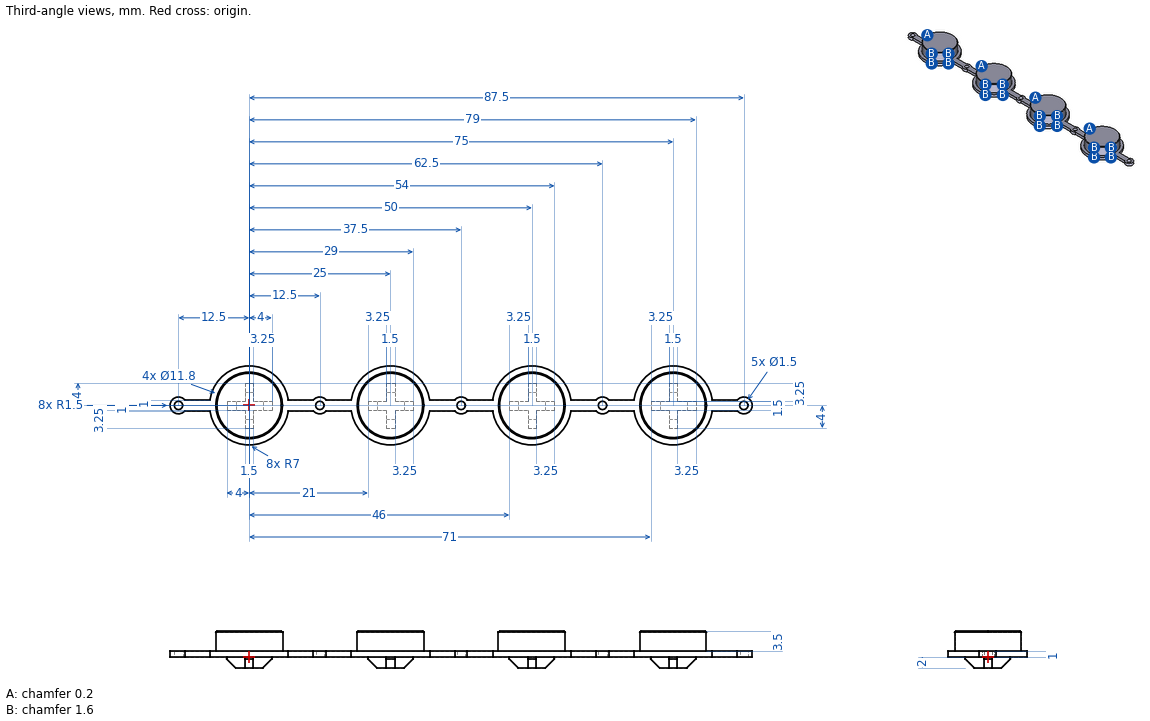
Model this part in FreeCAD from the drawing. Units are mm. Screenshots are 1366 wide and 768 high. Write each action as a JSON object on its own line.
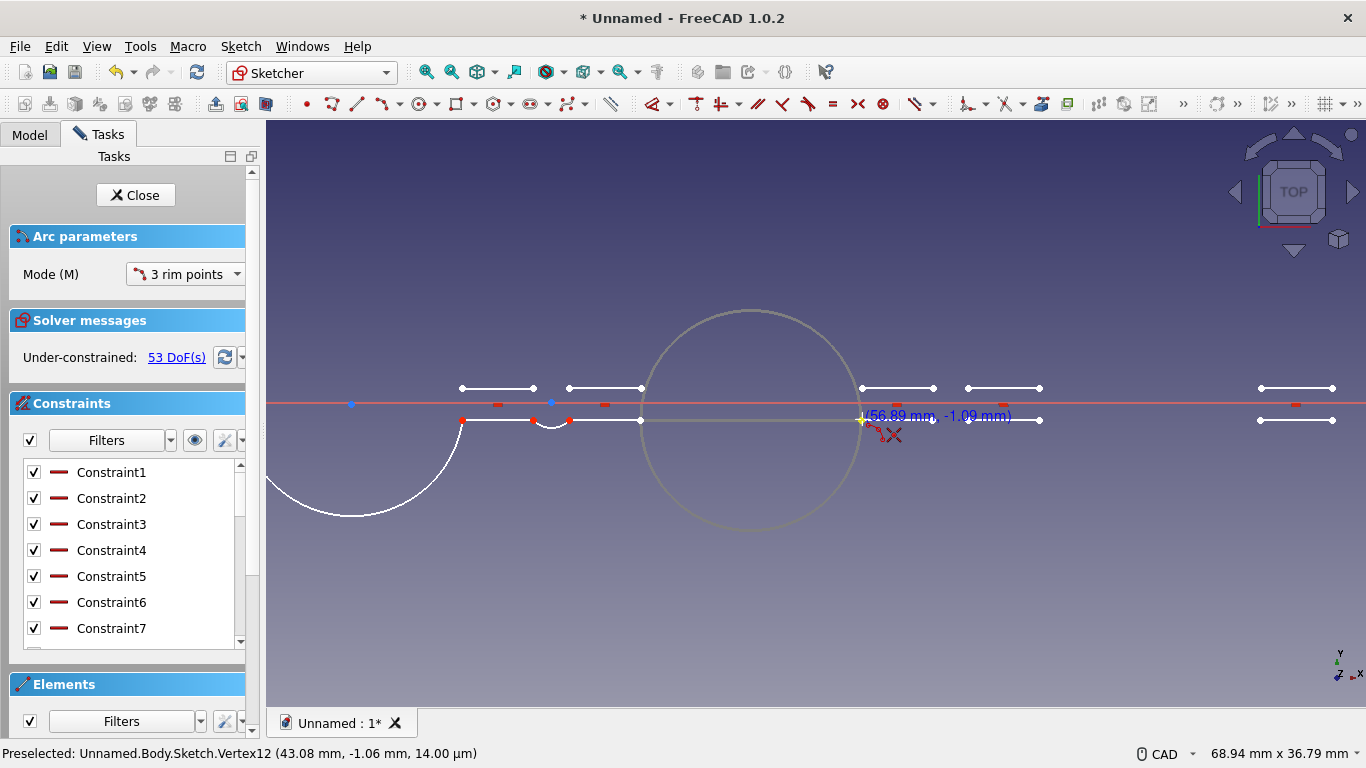
{"action": "left_click", "coordinate": [862, 420]}
{"action": "left_click", "coordinate": [751, 515]}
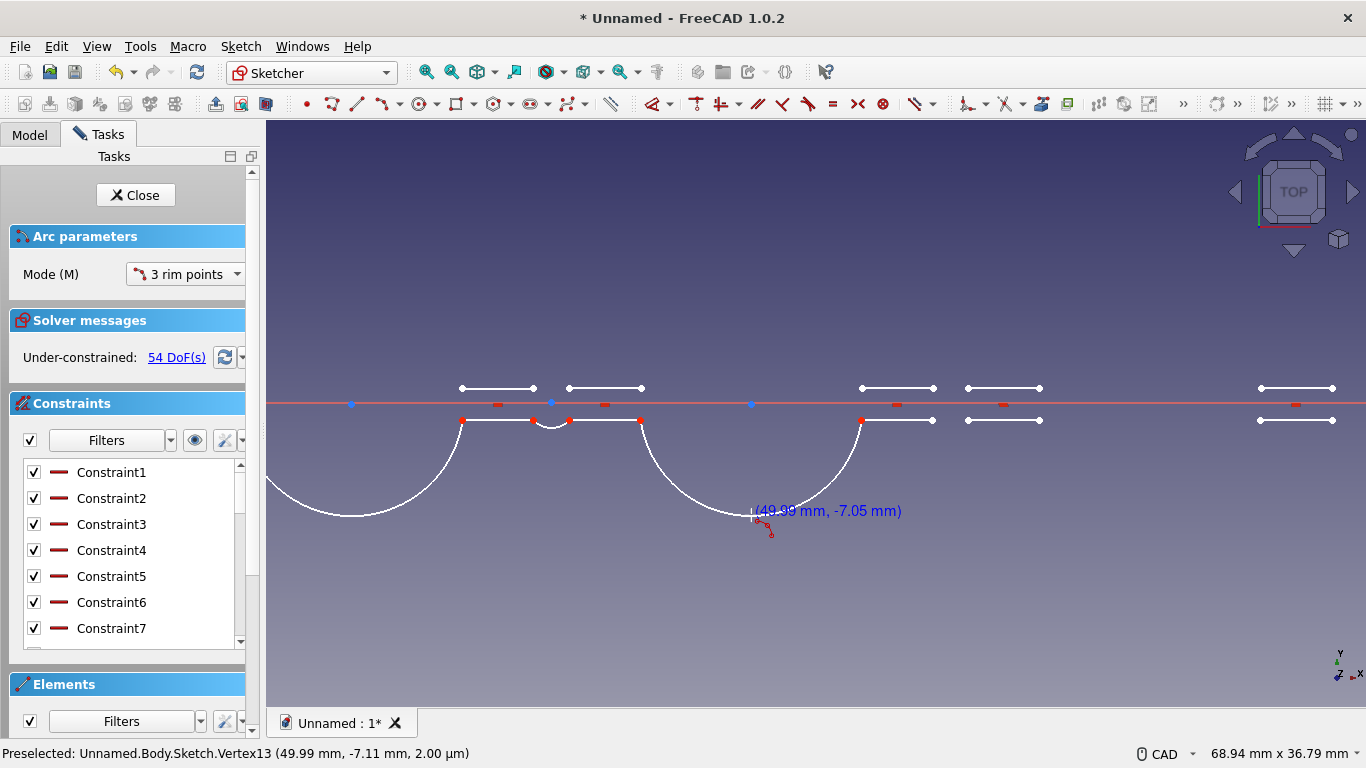
{"action": "left_click", "coordinate": [933, 420]}
{"action": "left_click", "coordinate": [969, 420]}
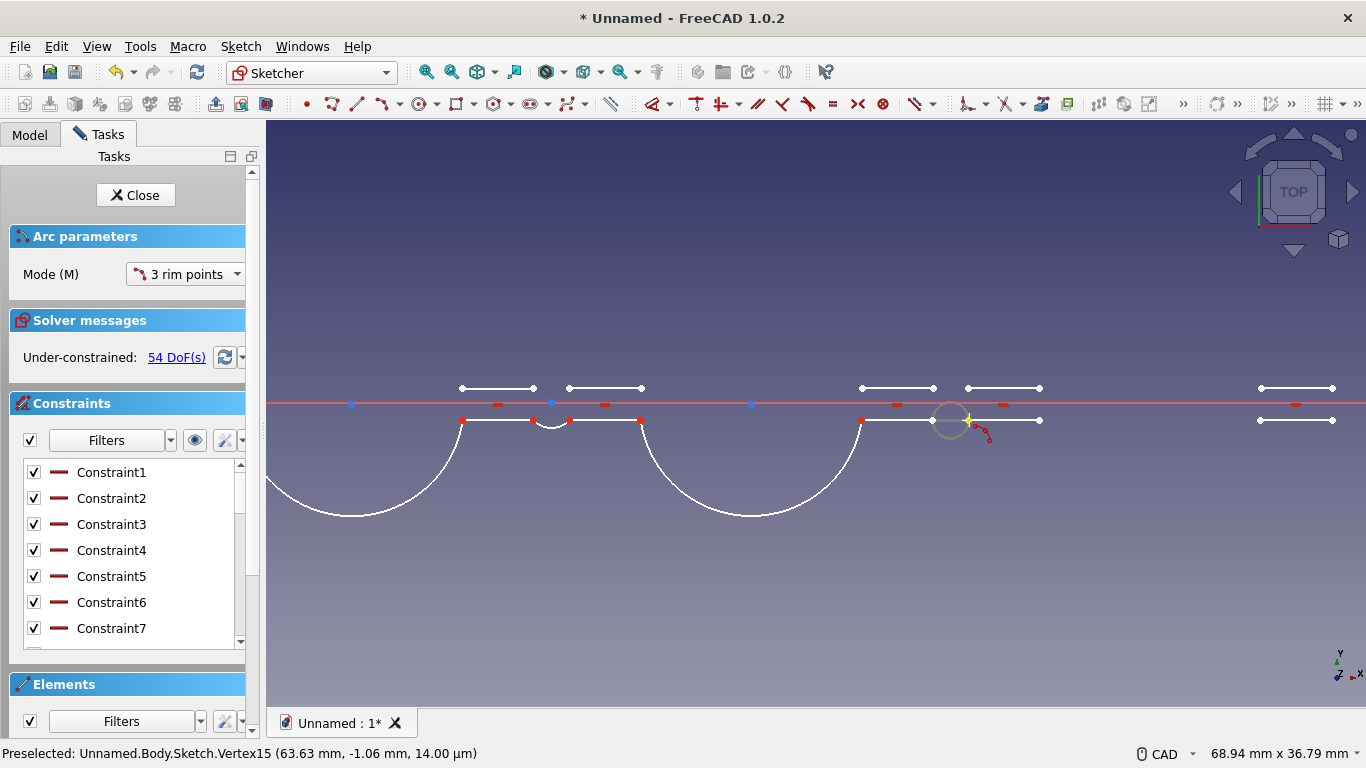
{"action": "scroll", "coordinate": [951, 427], "scroll_direction": "up", "scroll_amount": 4}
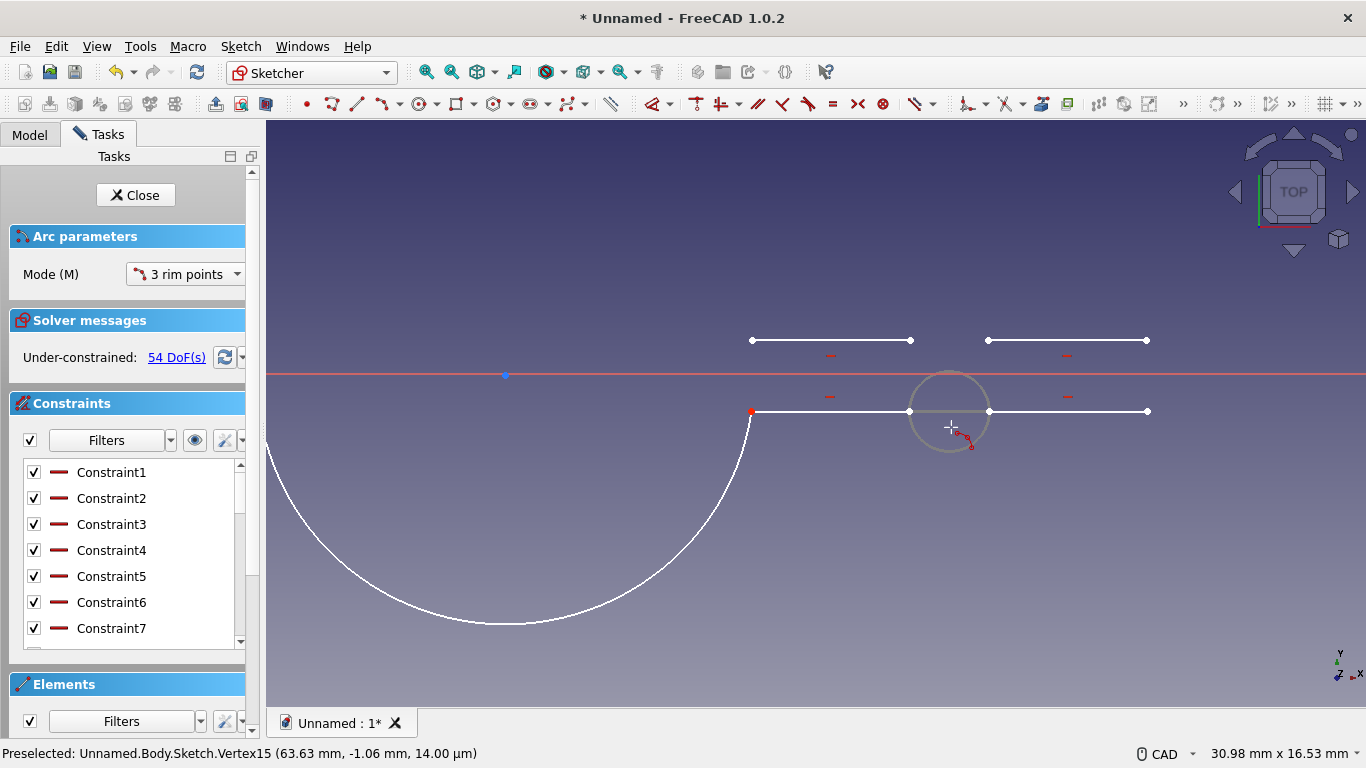
{"action": "left_click", "coordinate": [949, 427]}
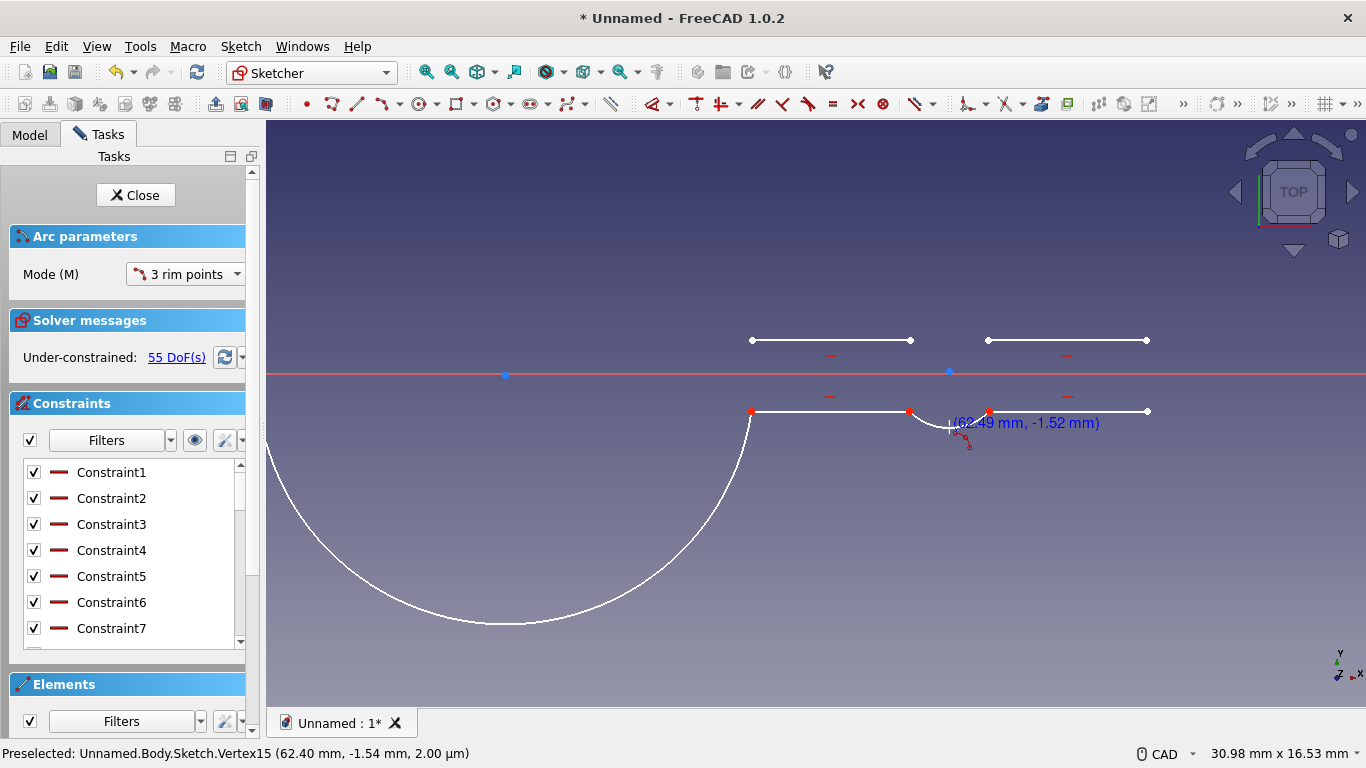
{"action": "left_click", "coordinate": [1147, 412]}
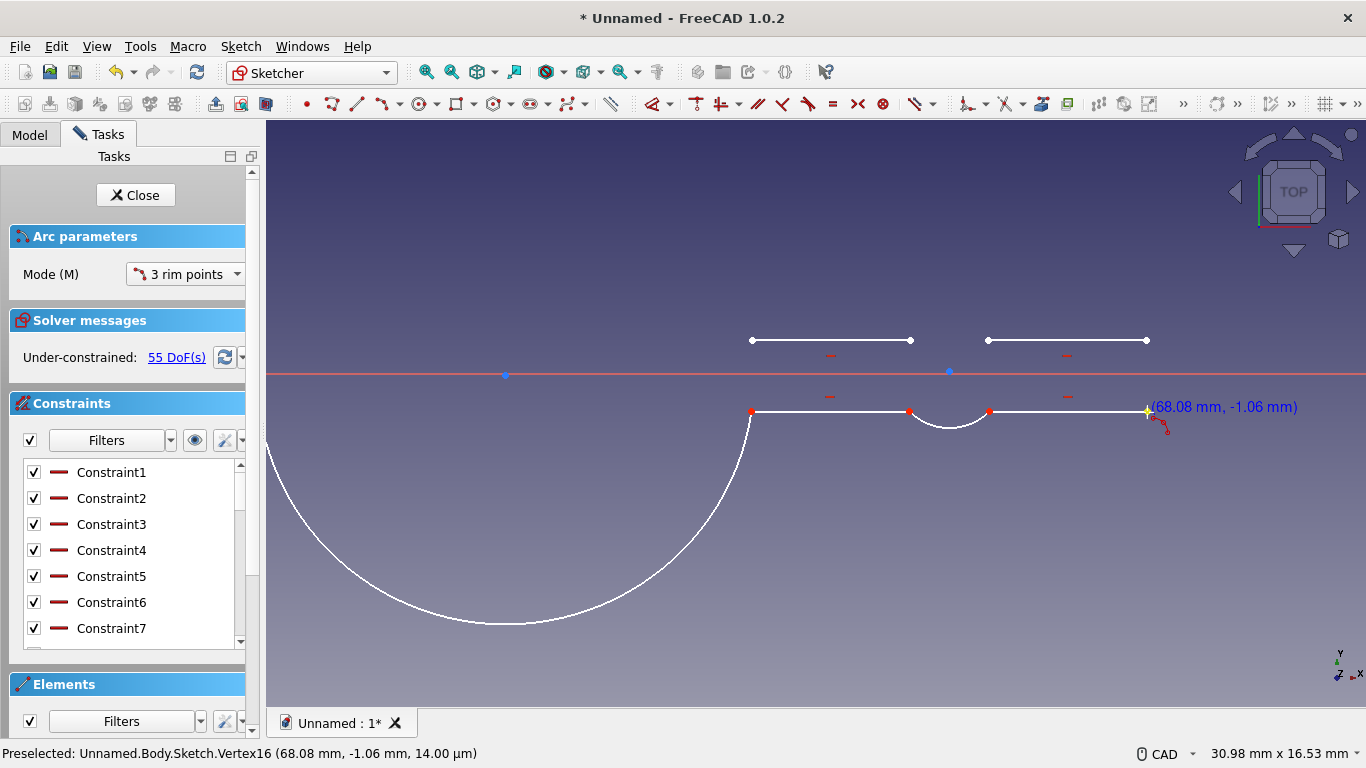
{"action": "scroll", "coordinate": [883, 421], "scroll_direction": "down", "scroll_amount": 9}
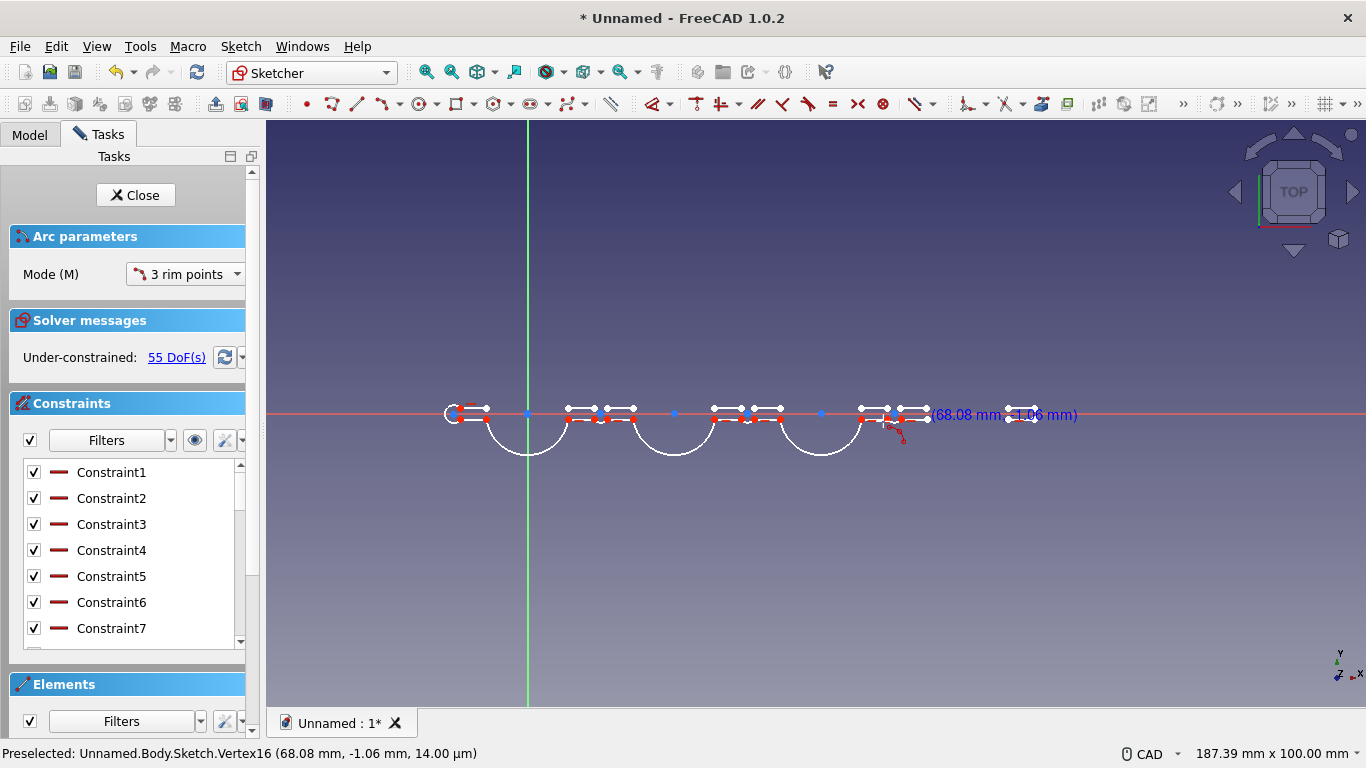
{"action": "scroll", "coordinate": [1008, 420], "scroll_direction": "up", "scroll_amount": 5}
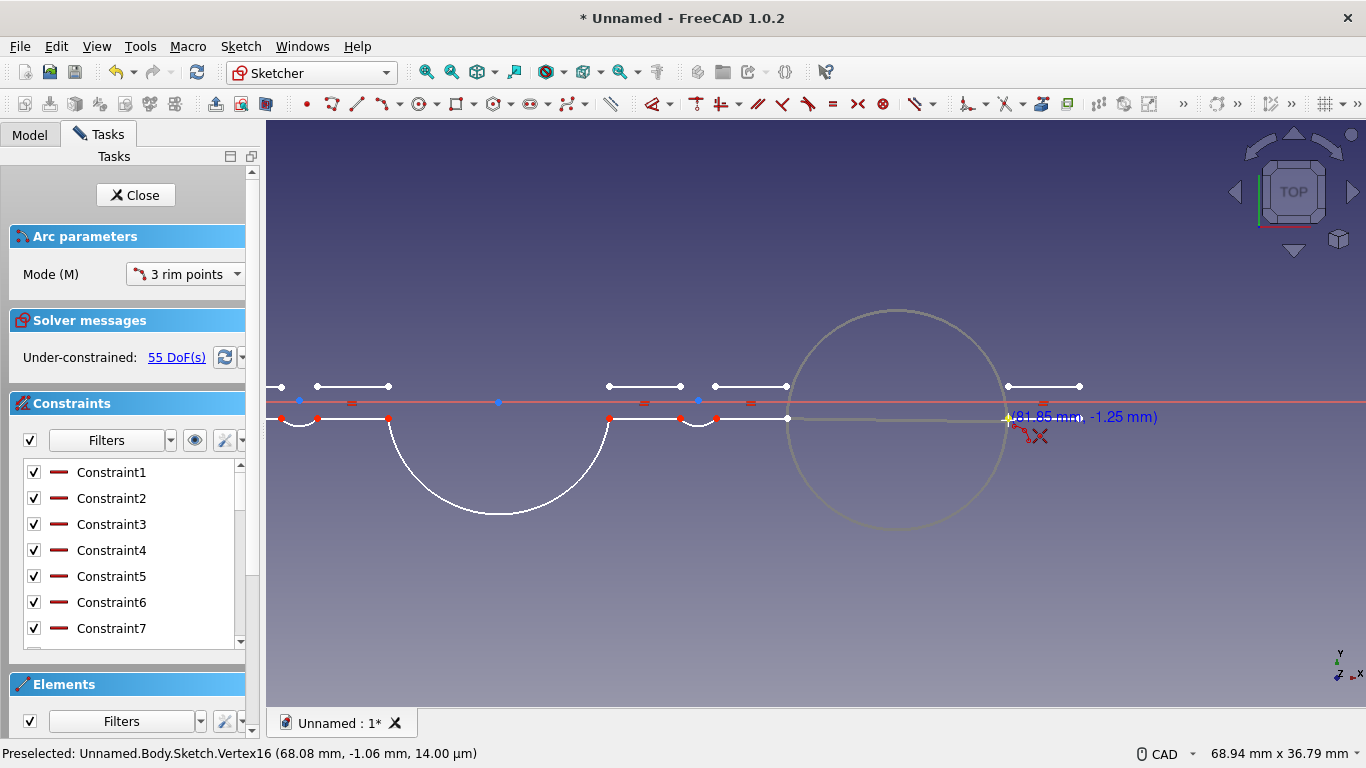
{"action": "left_click", "coordinate": [1008, 419]}
{"action": "left_click", "coordinate": [898, 514]}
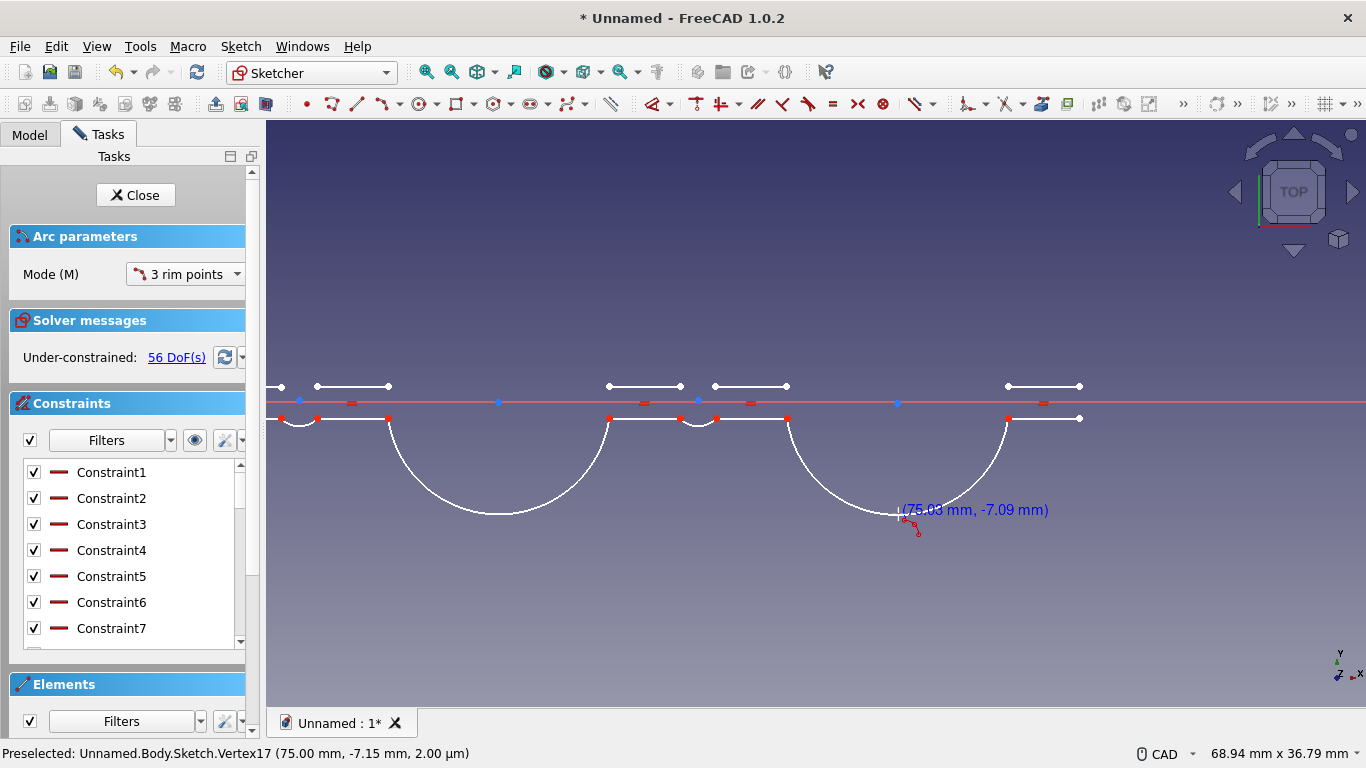
{"action": "left_click", "coordinate": [1080, 419]}
{"action": "left_click", "coordinate": [1080, 387]}
{"action": "left_click", "coordinate": [1111, 422]}